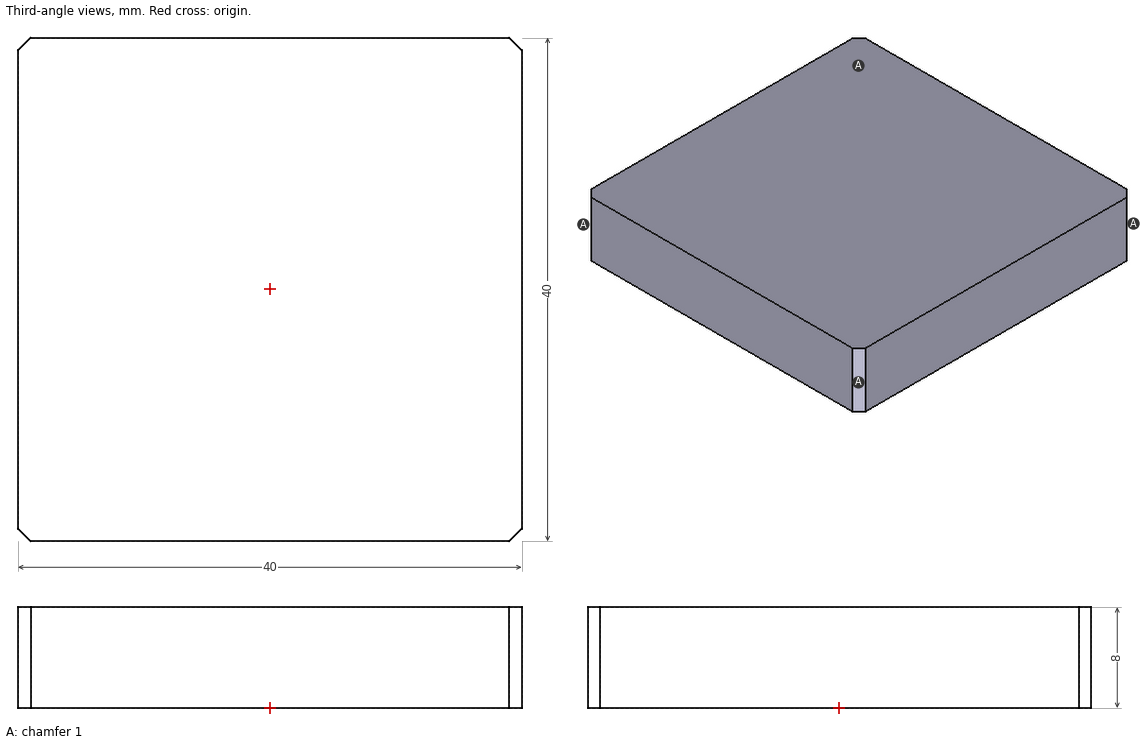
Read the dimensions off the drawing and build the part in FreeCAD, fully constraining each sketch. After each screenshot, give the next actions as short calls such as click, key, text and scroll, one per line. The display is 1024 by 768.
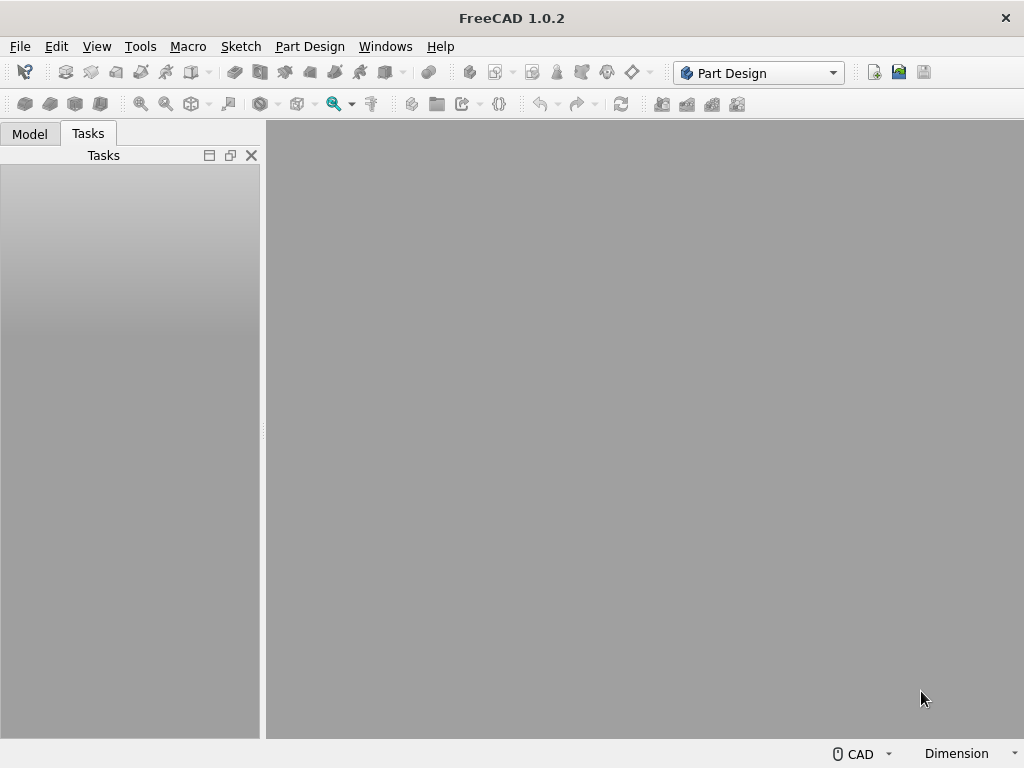
click(874, 72)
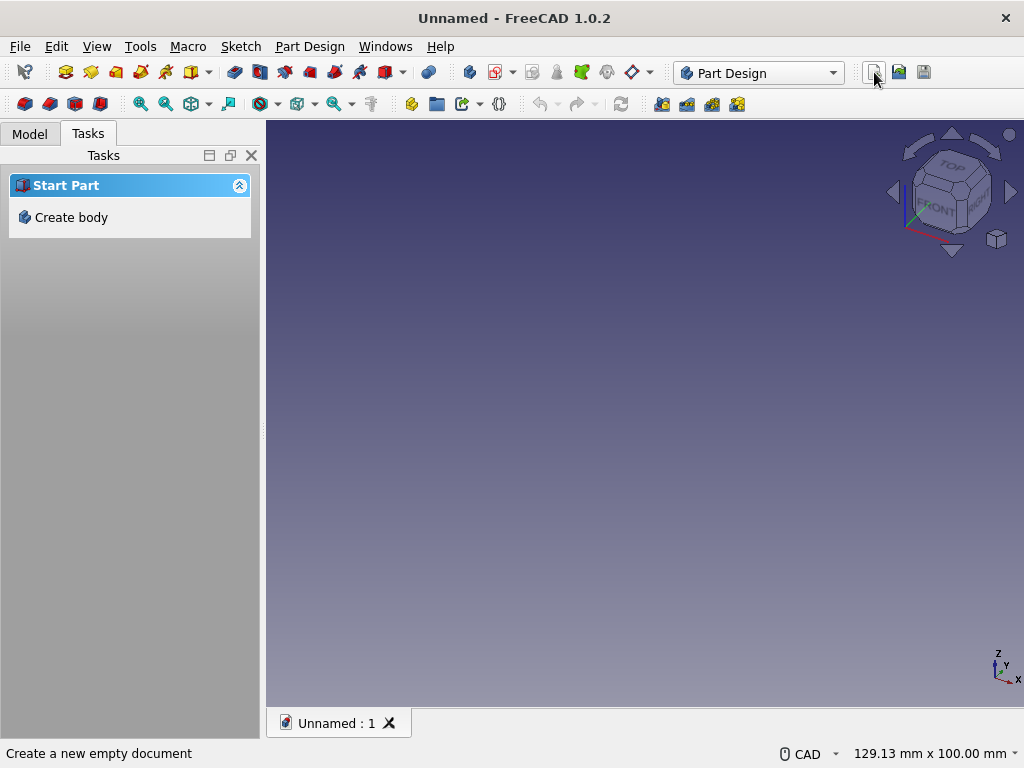
click(494, 72)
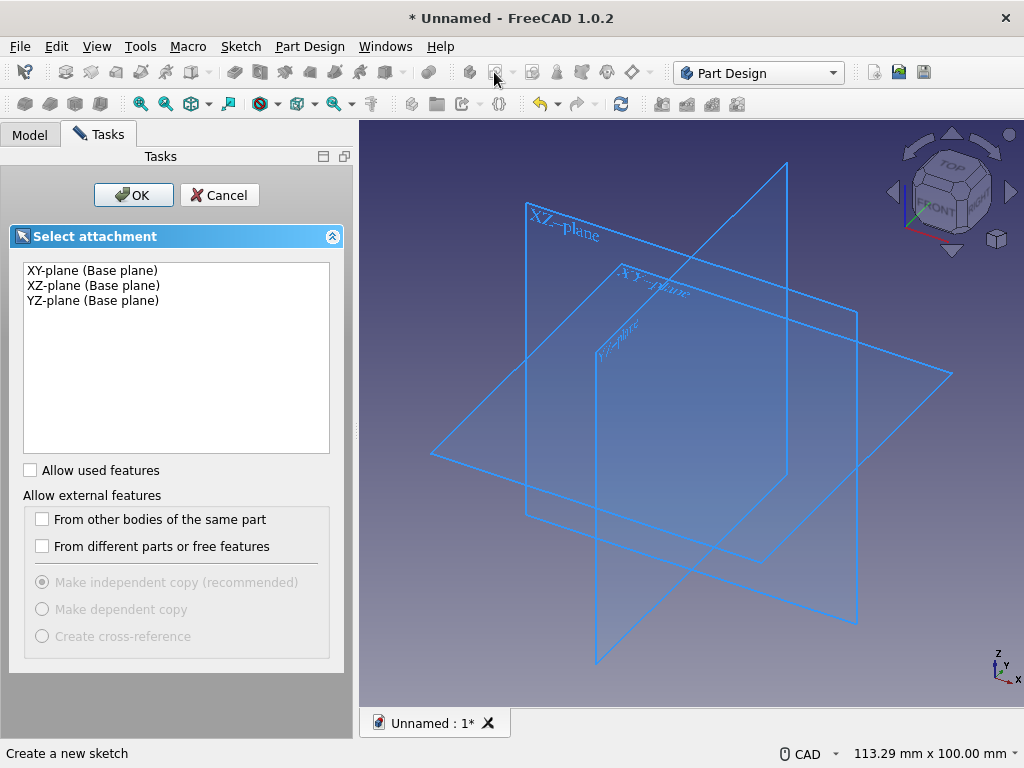
click(84, 270)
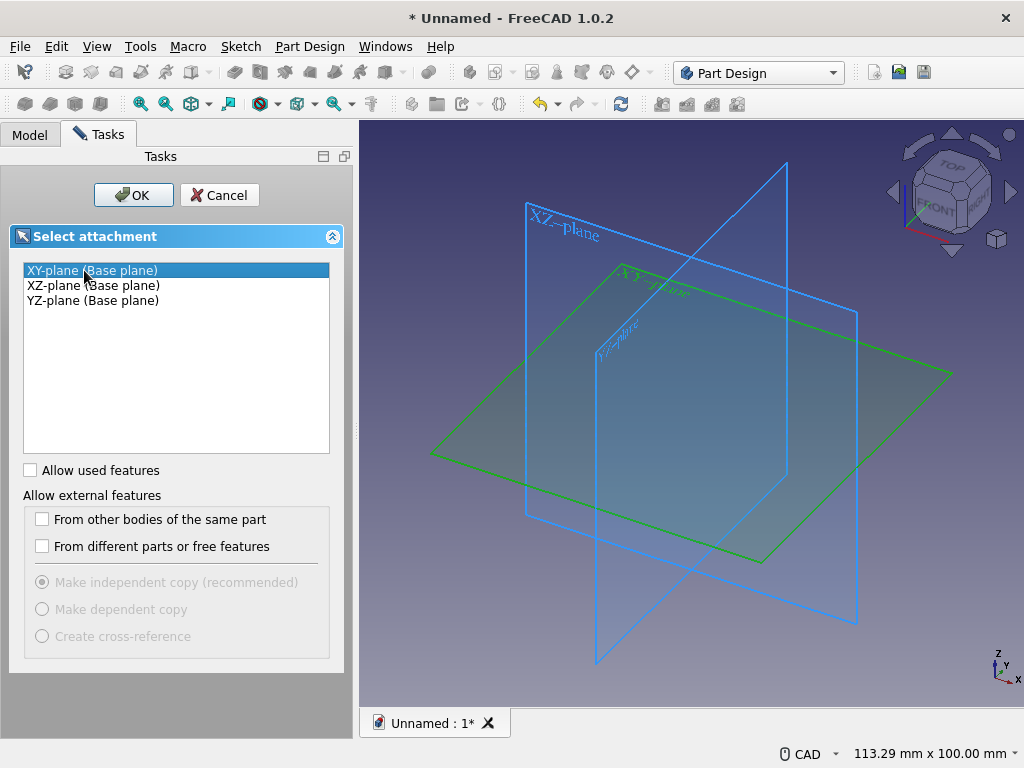
click(134, 195)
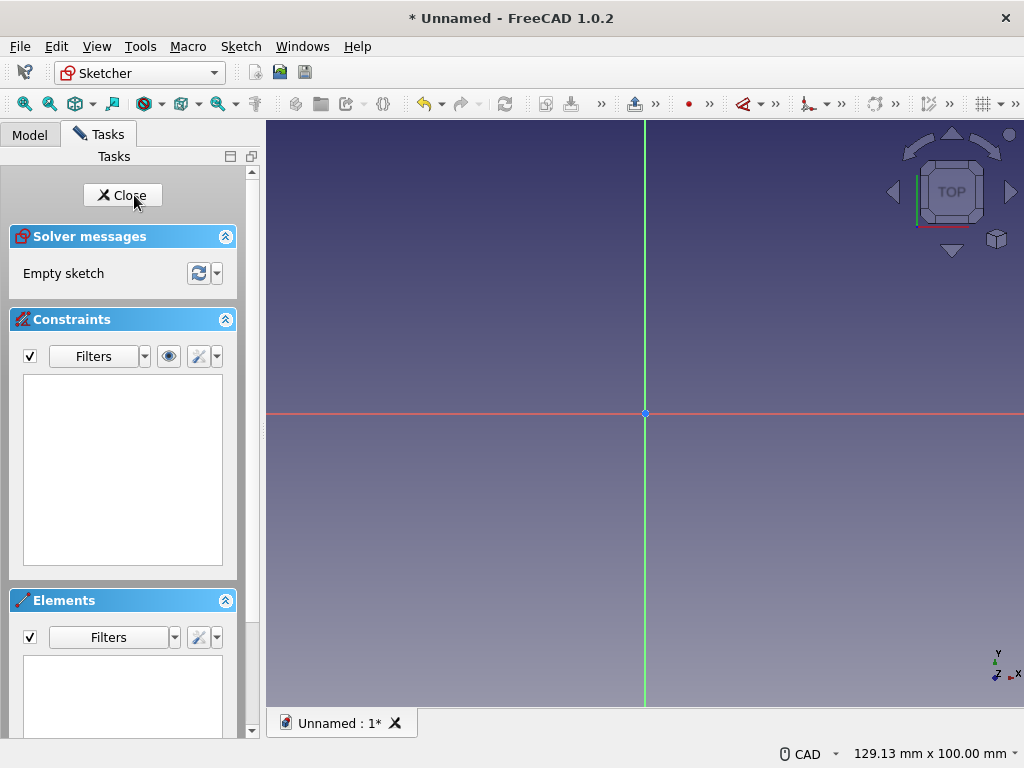
scroll(784, 413, up, 2)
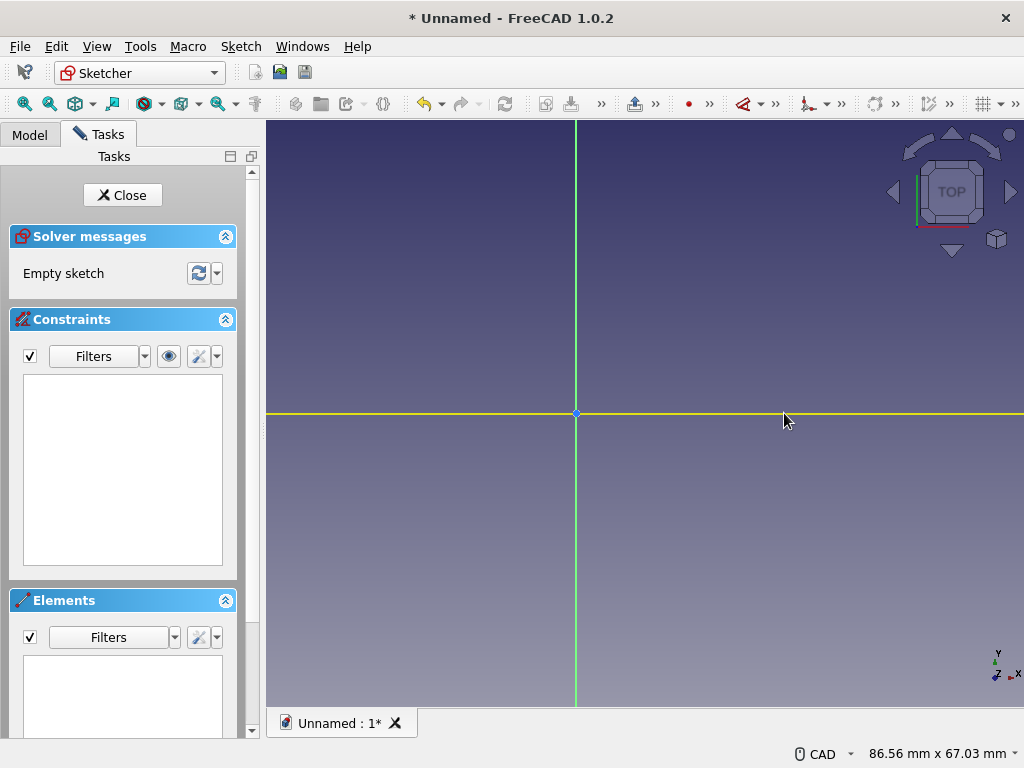
key(g)
key(v)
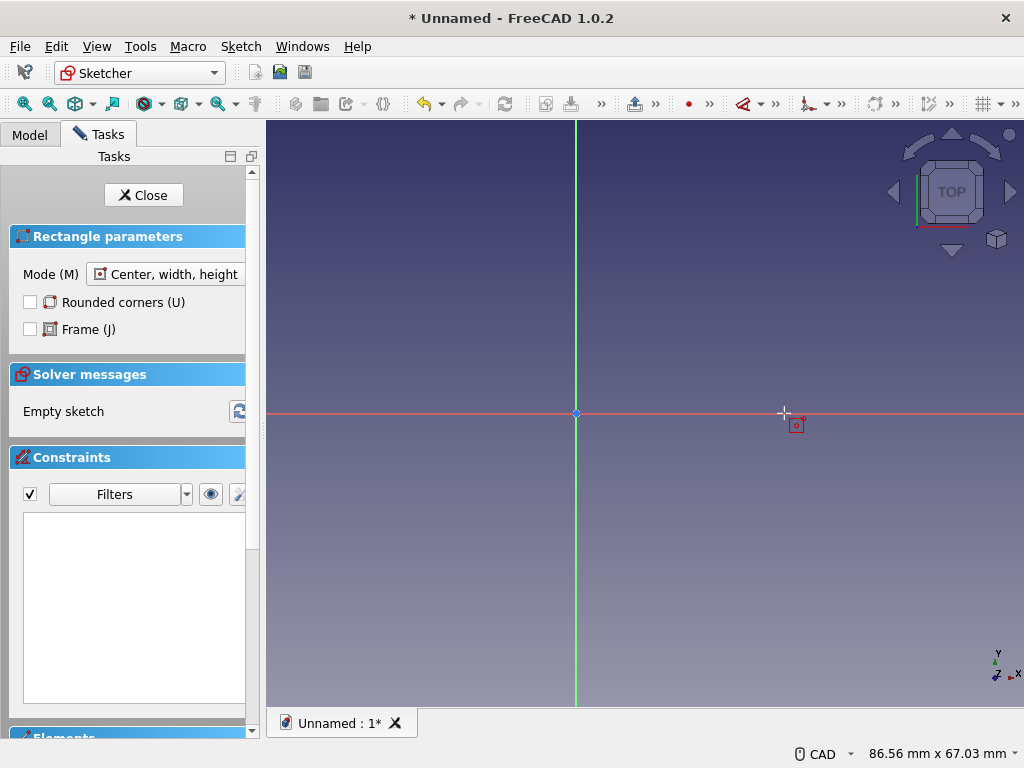
click(576, 414)
click(751, 238)
key(Escape)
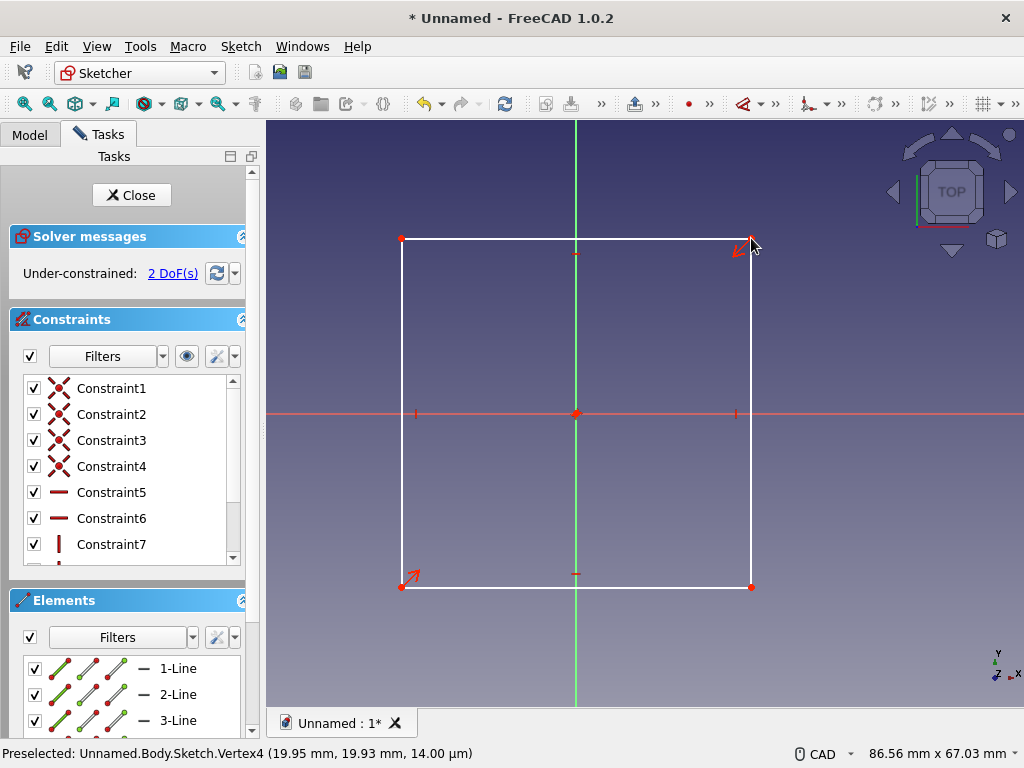
click(742, 104)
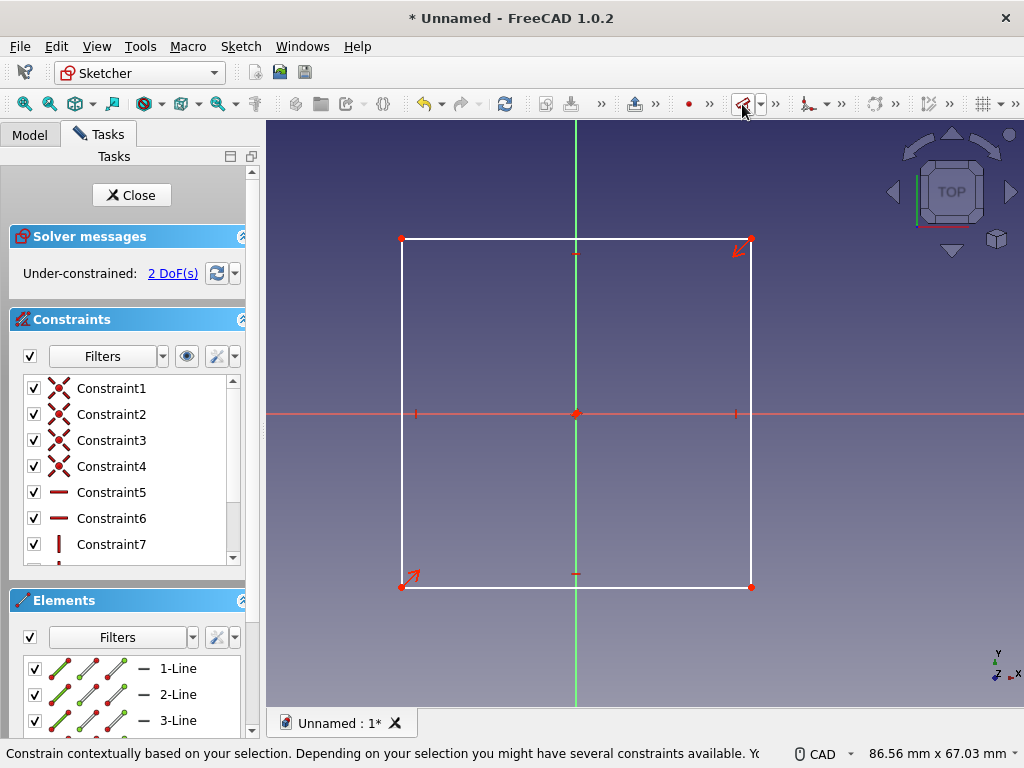
click(506, 588)
click(496, 622)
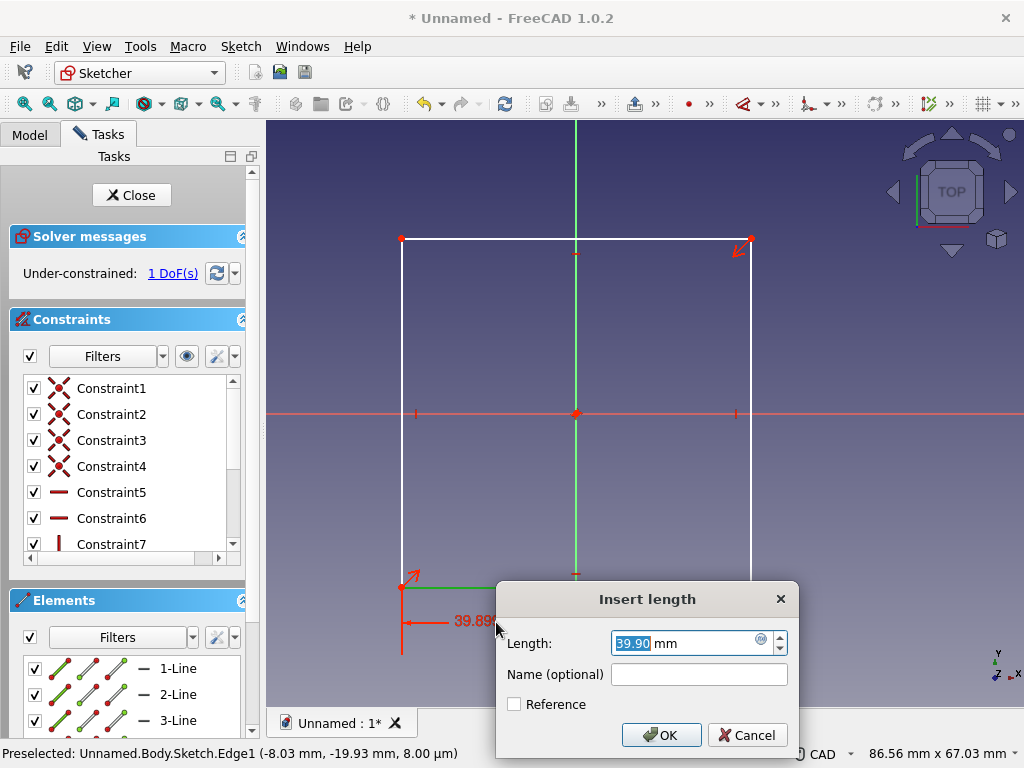
text(40)
key(Return)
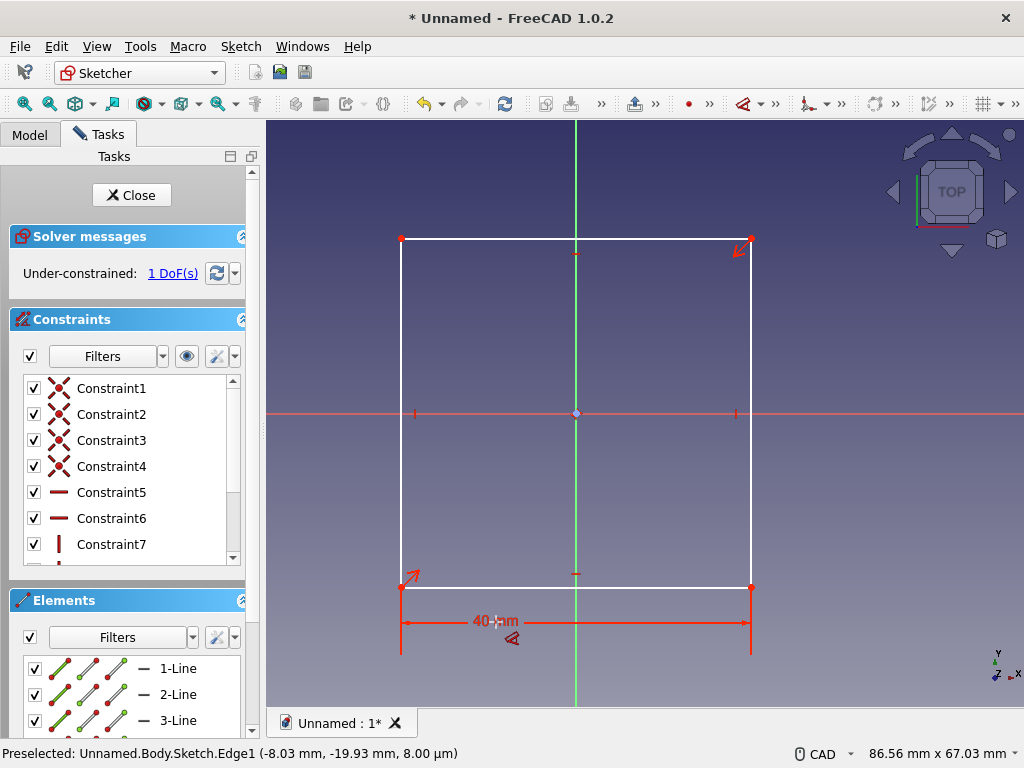
click(751, 483)
click(785, 333)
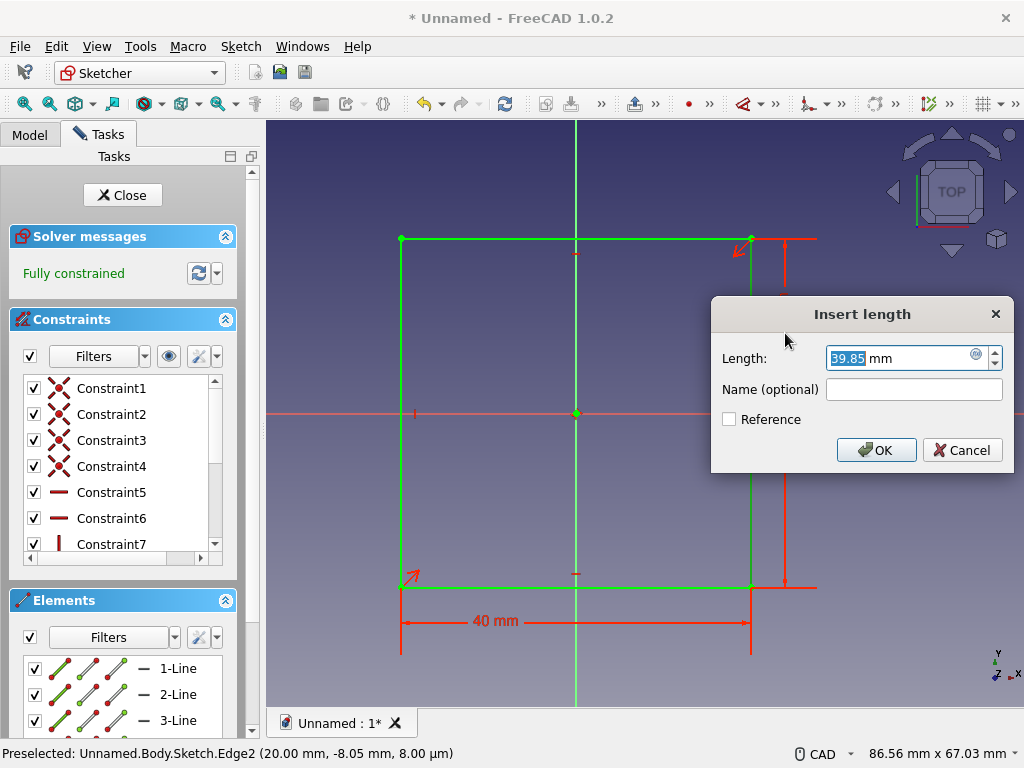
text(40)
key(Return)
key(Escape)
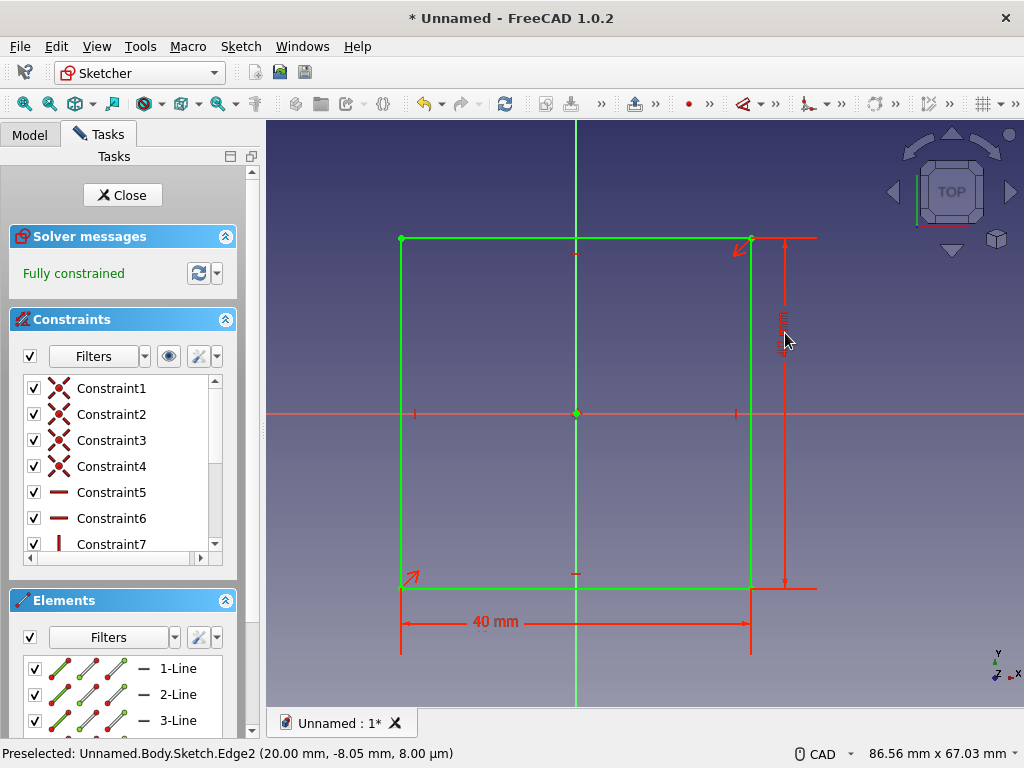
click(123, 195)